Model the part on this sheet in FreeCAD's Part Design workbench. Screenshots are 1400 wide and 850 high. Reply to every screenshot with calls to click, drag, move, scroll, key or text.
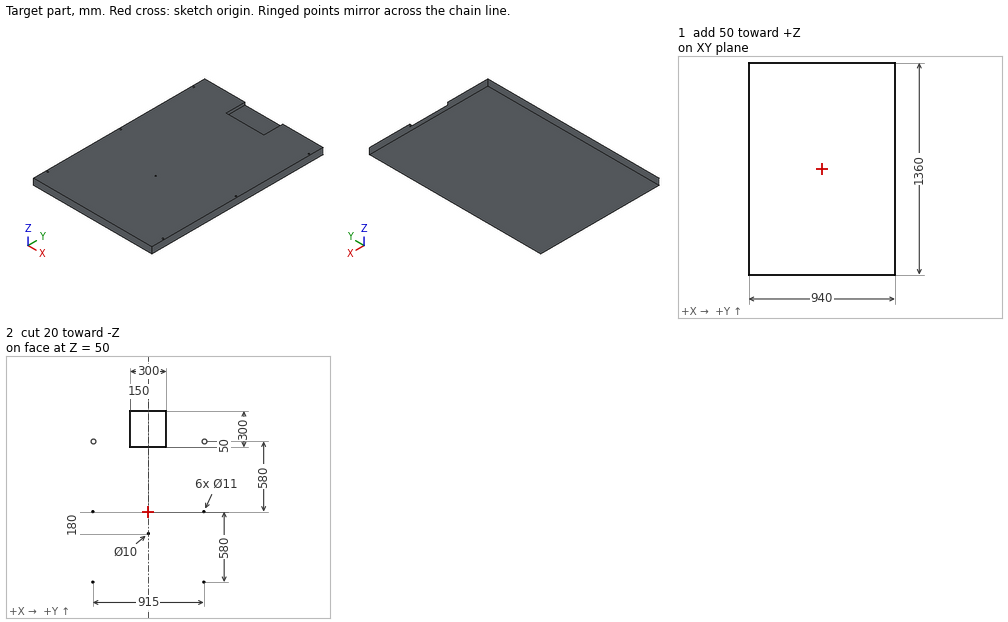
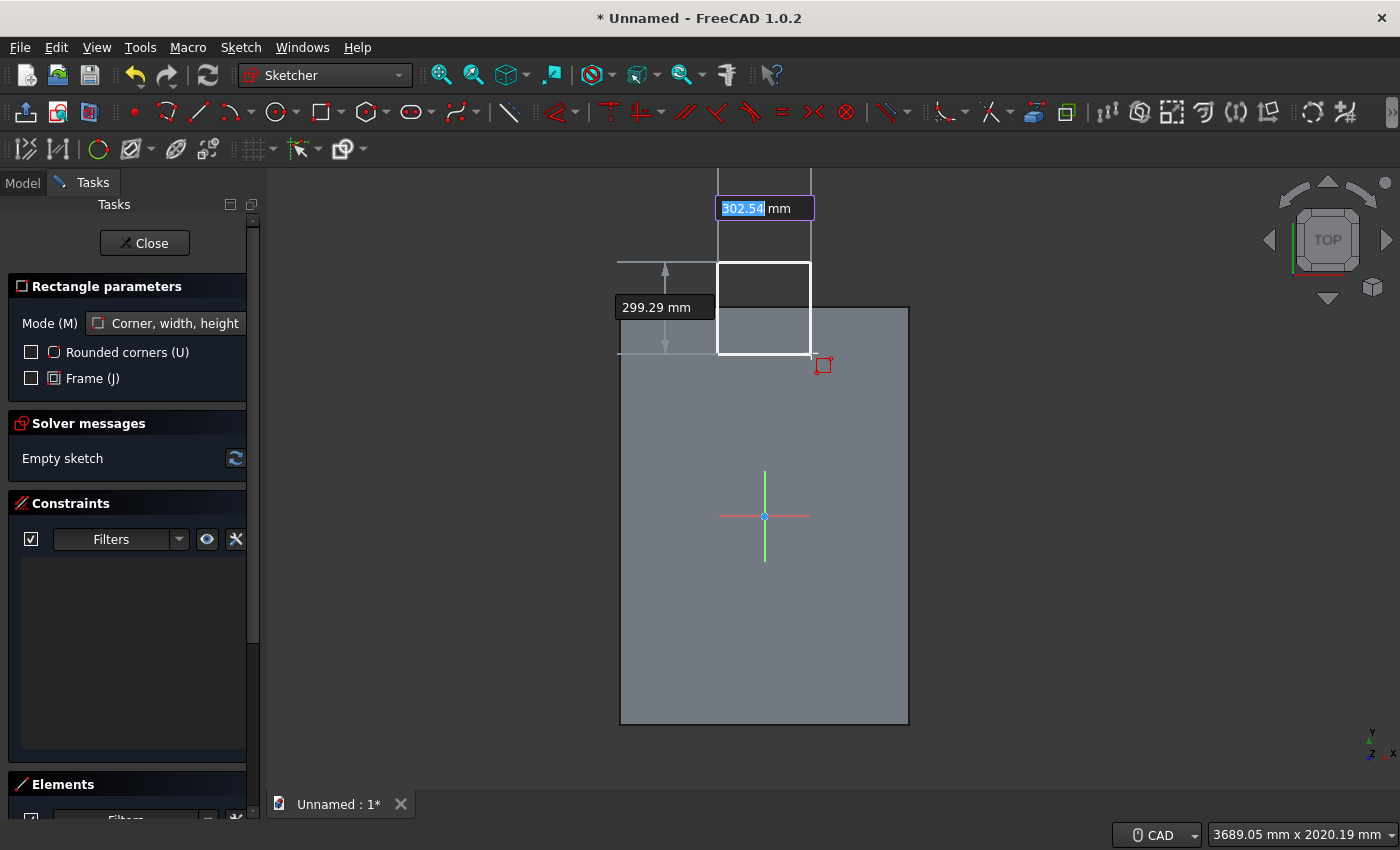
text(300)
key(Tab)
text(300)
key(Return)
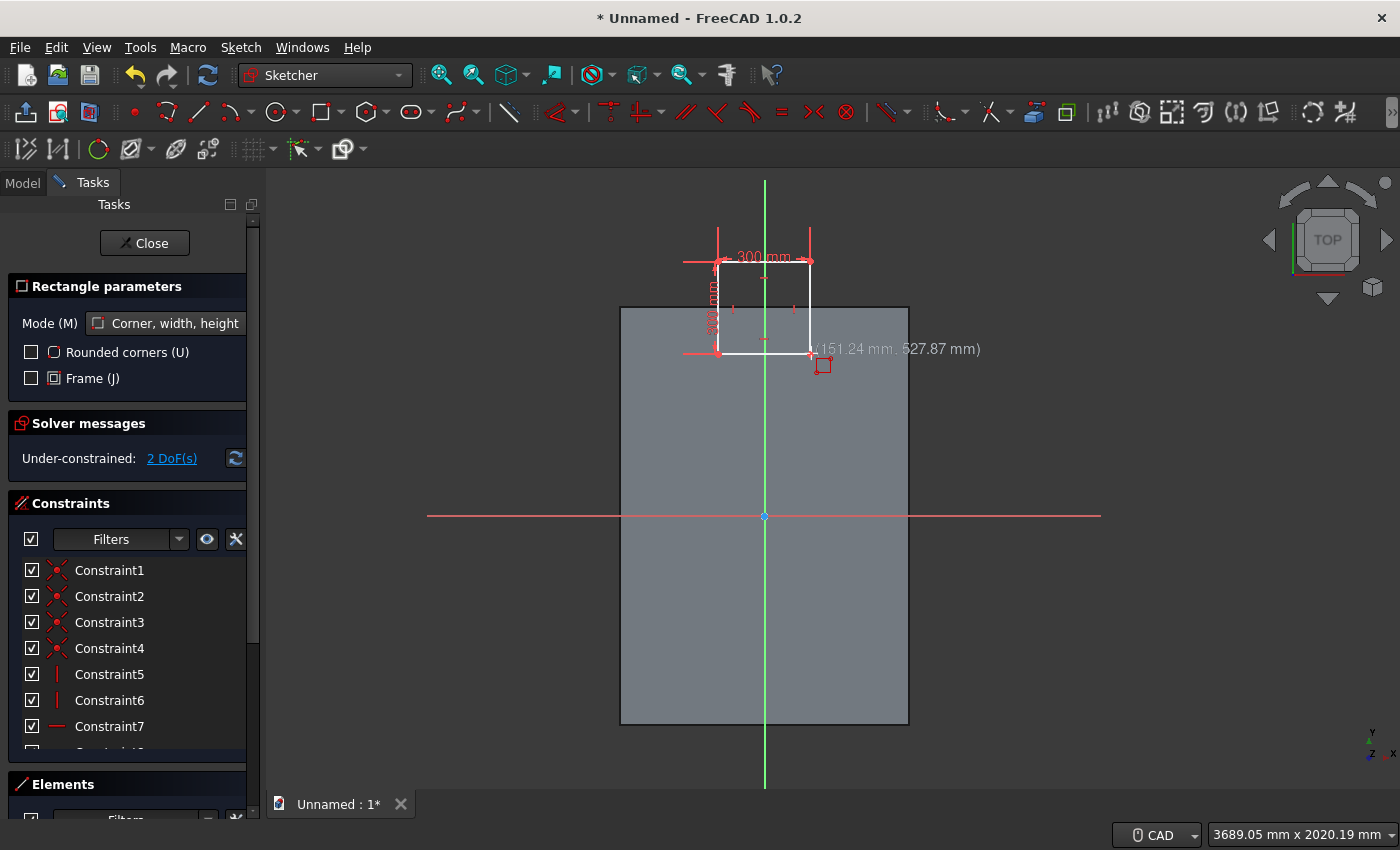
click(276, 112)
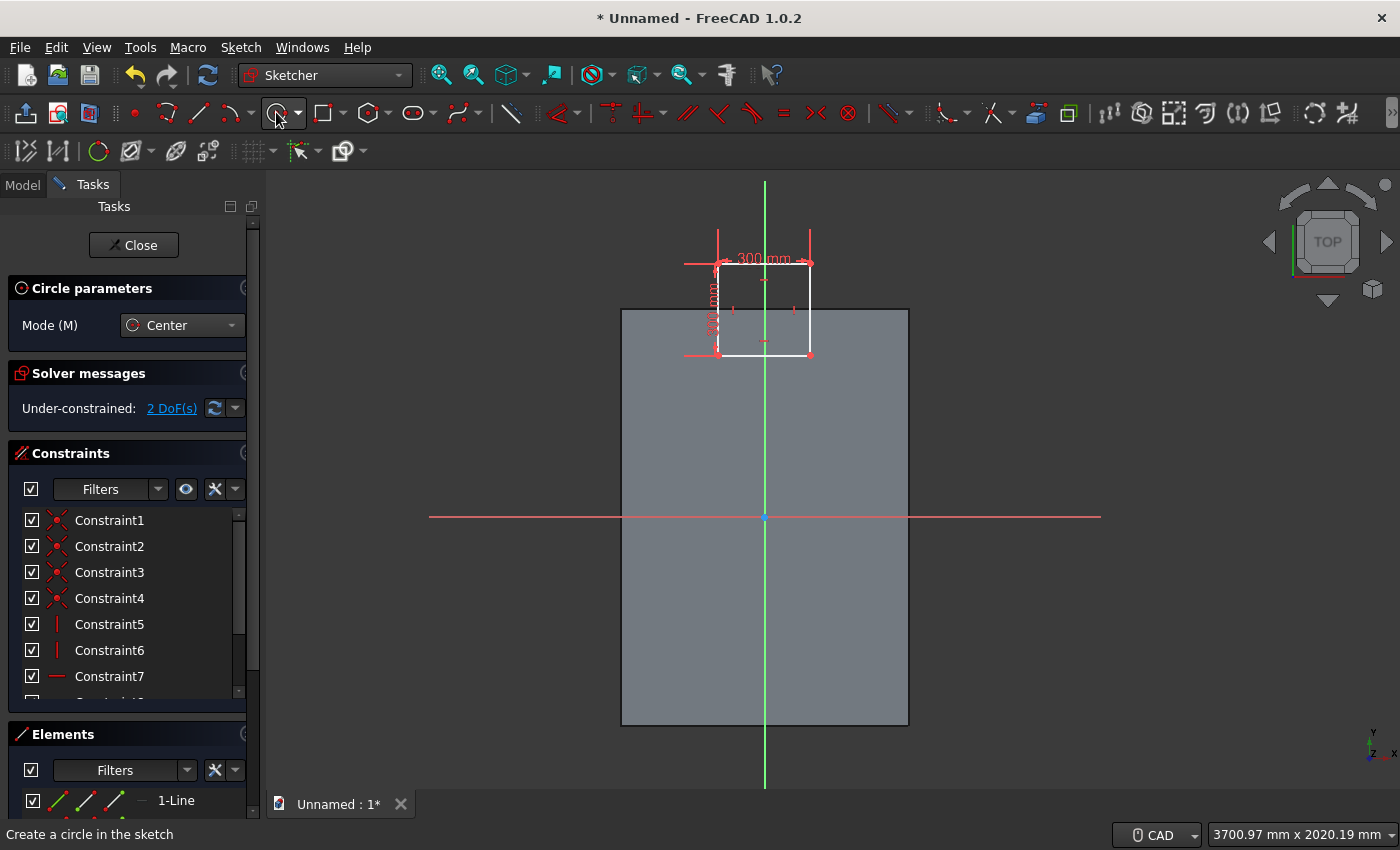
scroll(765, 572, up, 14)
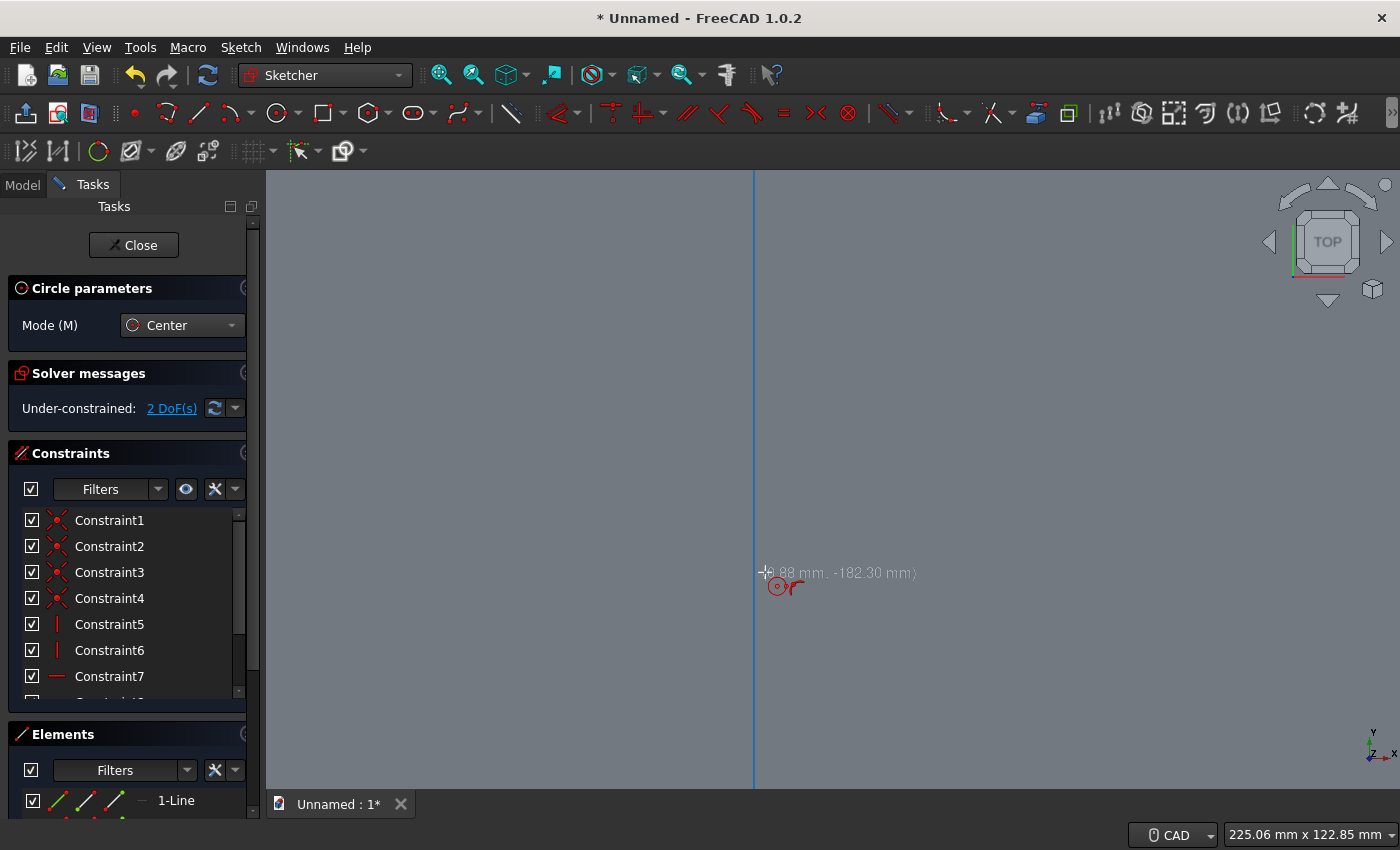
scroll(765, 572, down, 14)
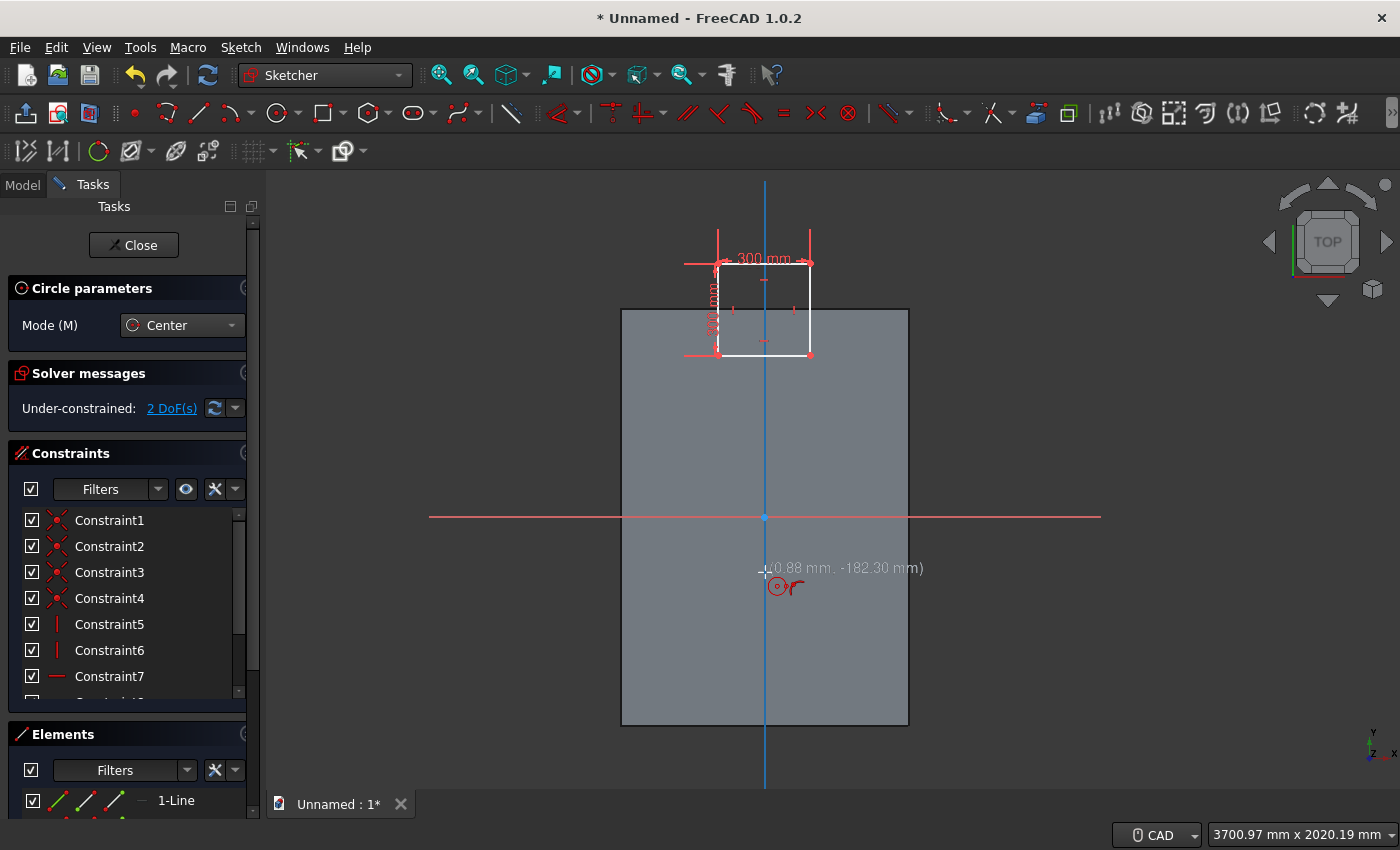
click(765, 572)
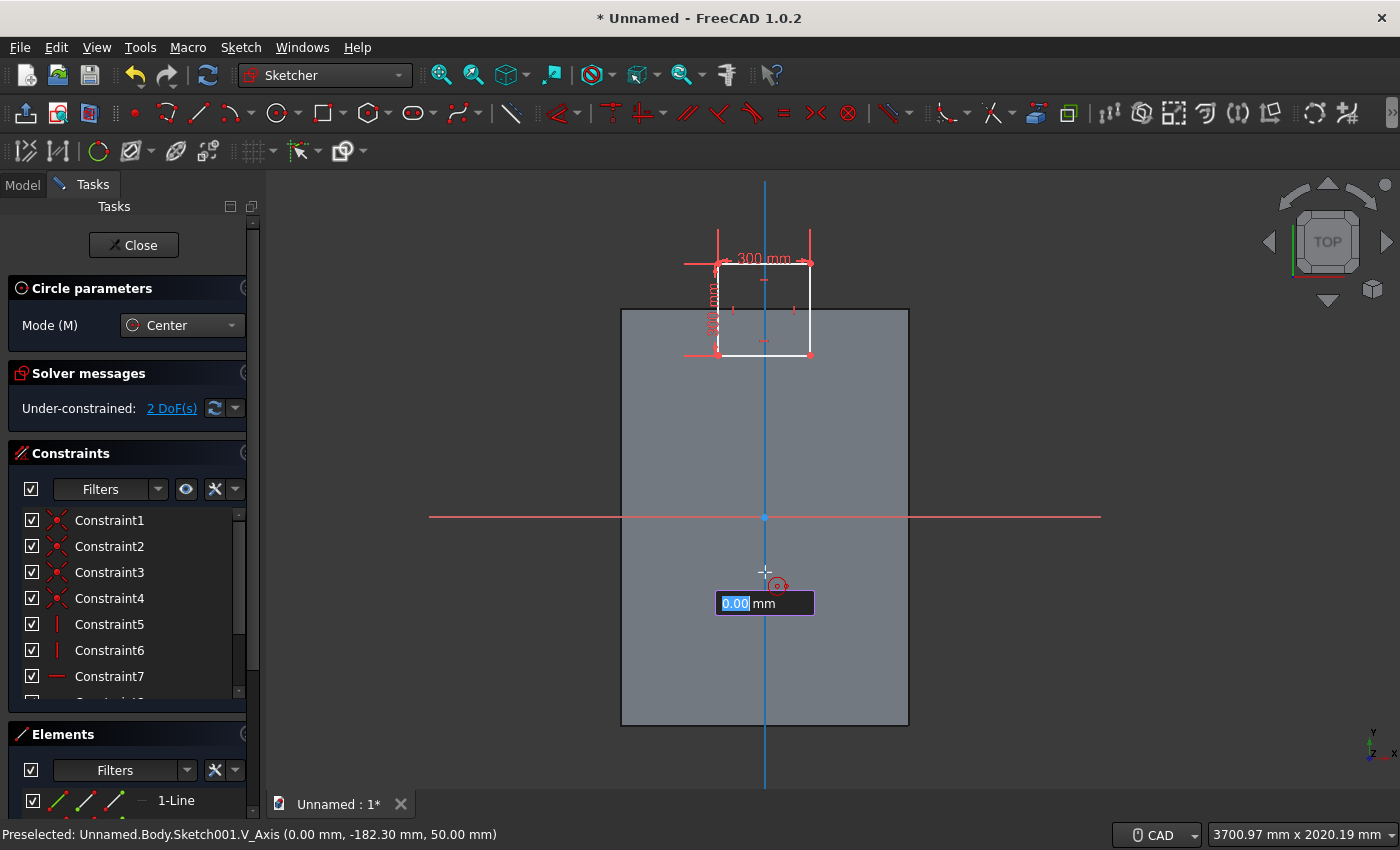
scroll(766, 572, up, 13)
move(763, 561)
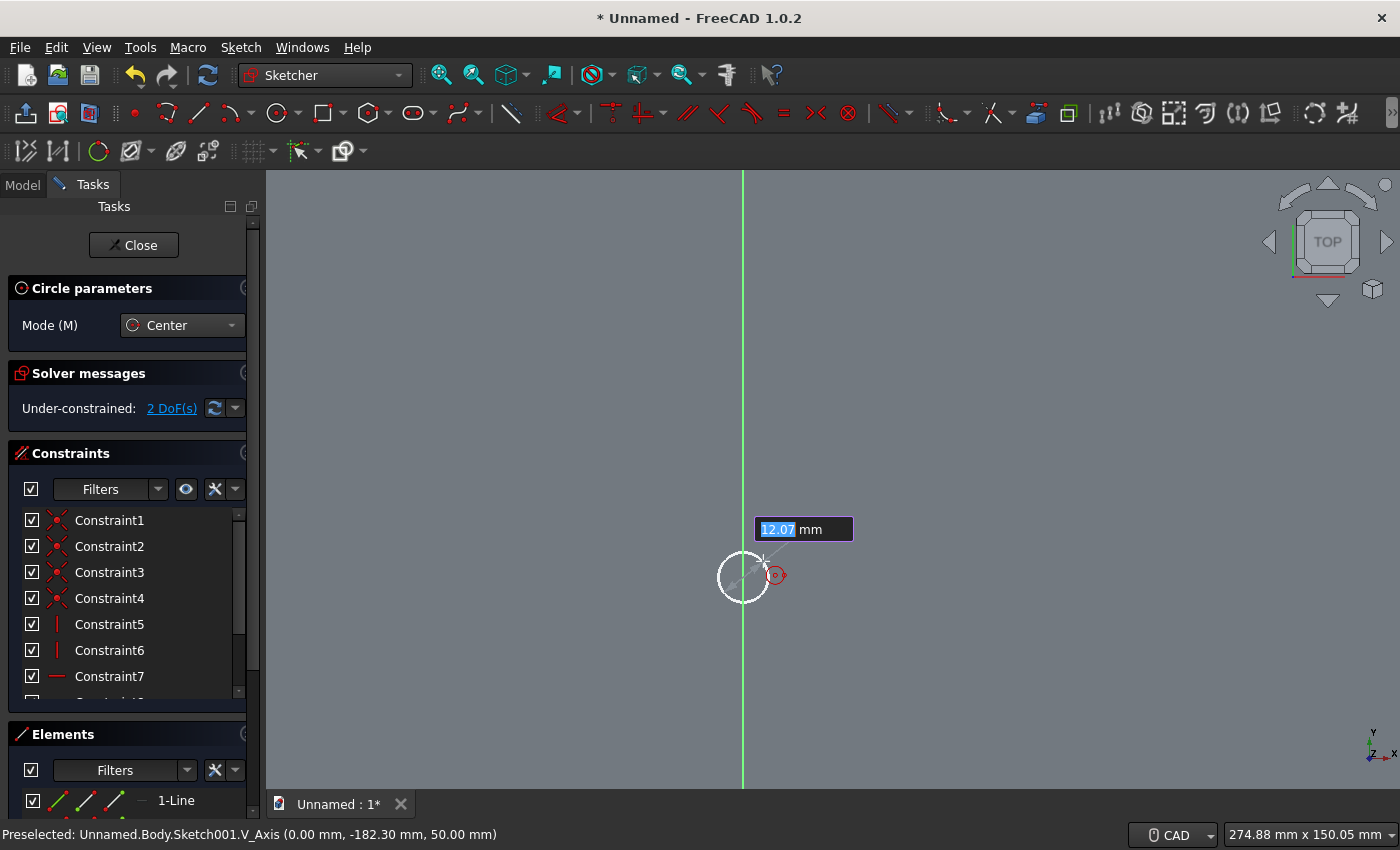
text(10)
key(Return)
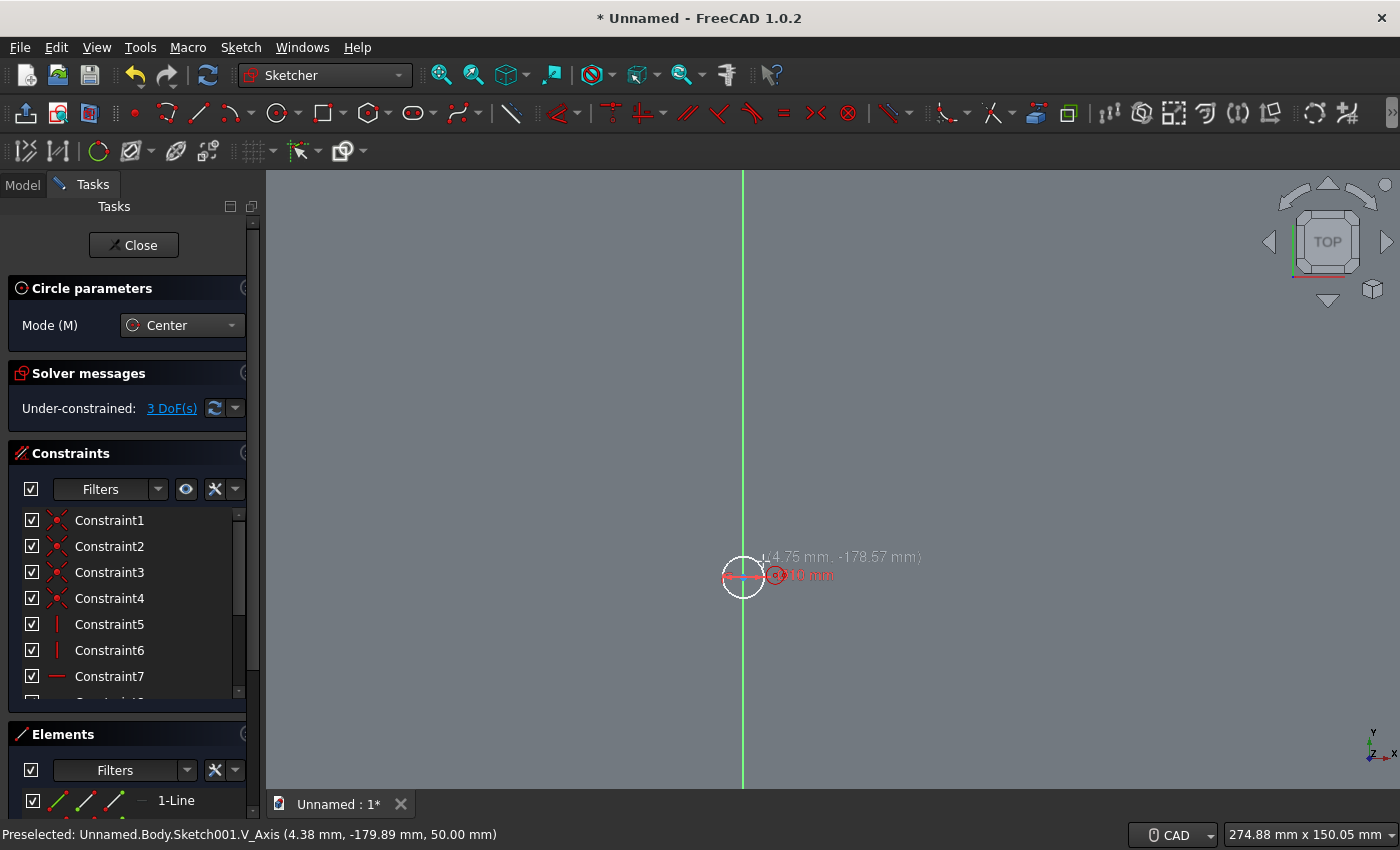
scroll(766, 572, down, 13)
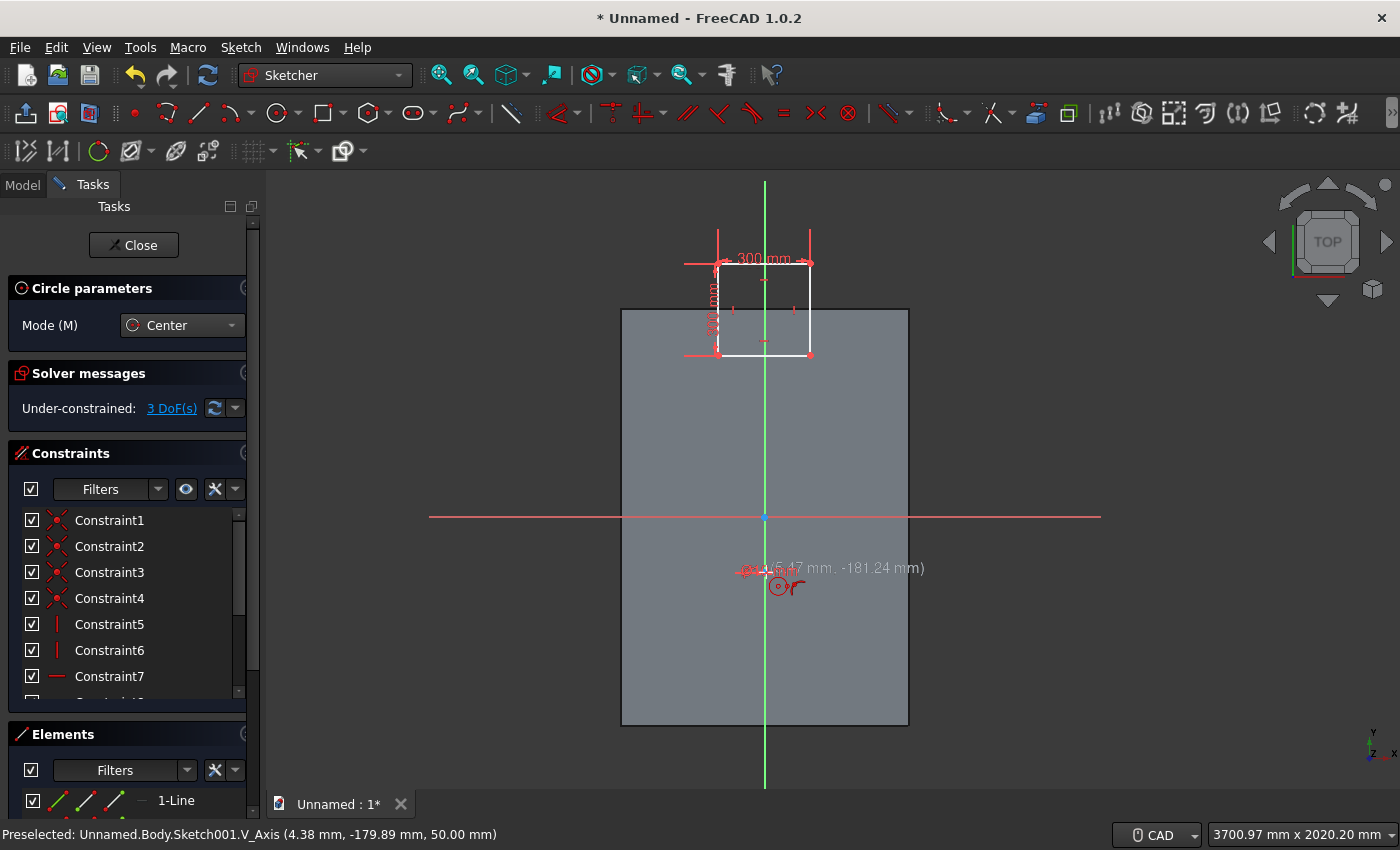
scroll(905, 695, up, 13)